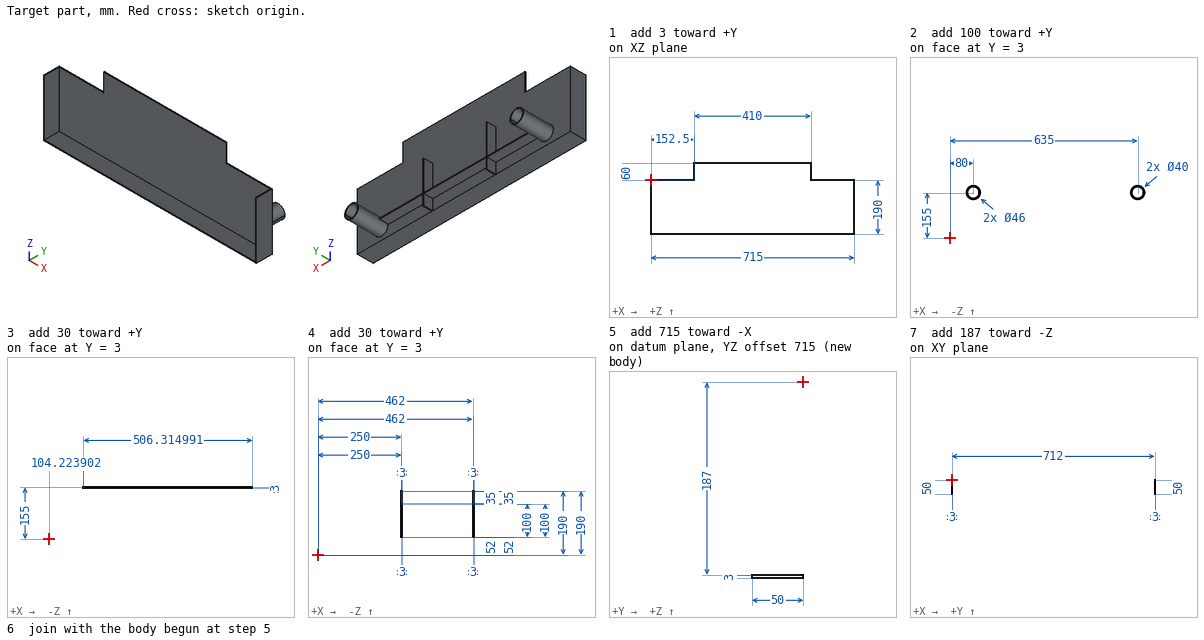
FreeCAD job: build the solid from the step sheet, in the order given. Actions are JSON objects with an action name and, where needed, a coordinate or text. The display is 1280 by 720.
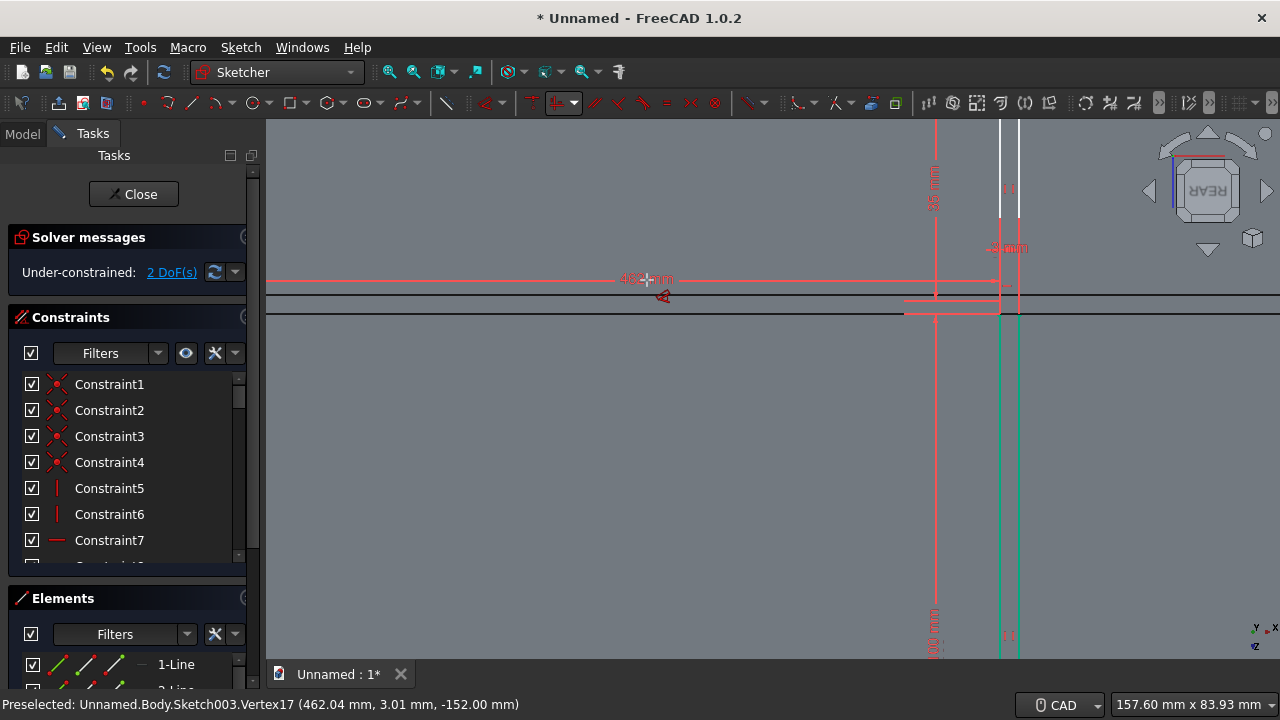
{"action": "scroll", "coordinate": [1003, 315], "scroll_direction": "down", "scroll_amount": 8}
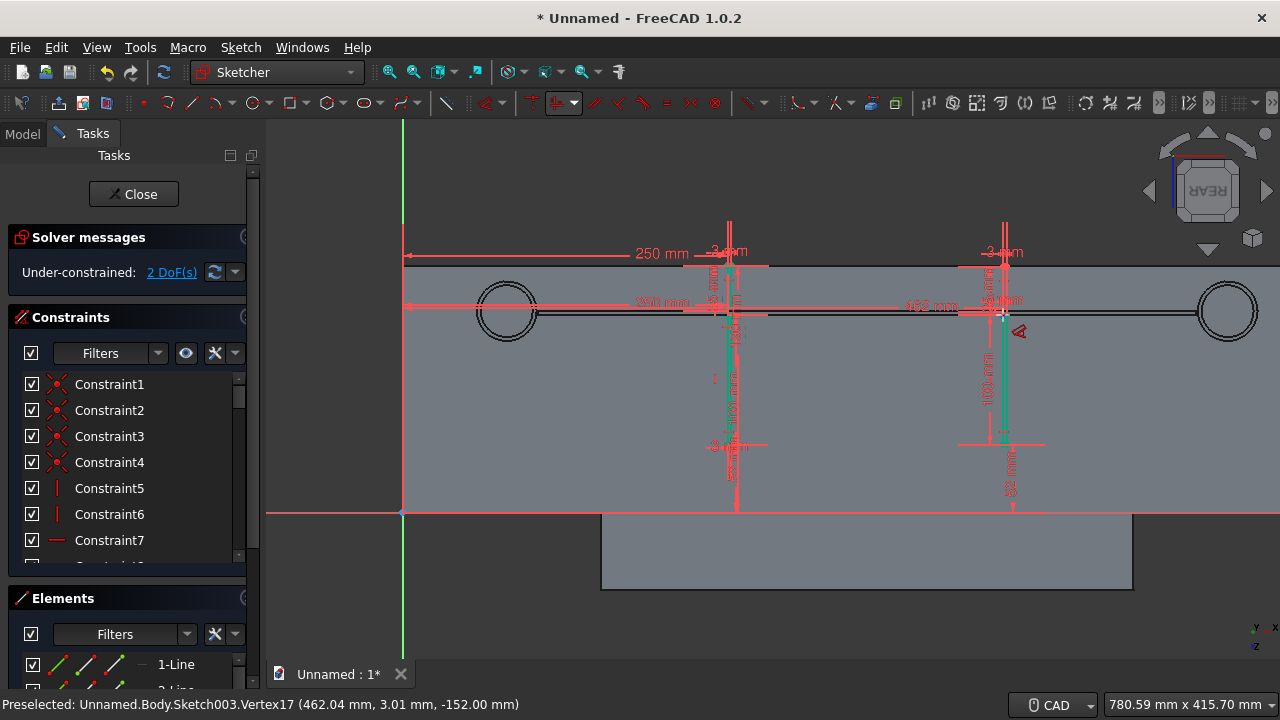
{"action": "scroll", "coordinate": [1003, 267], "scroll_direction": "up", "scroll_amount": 6}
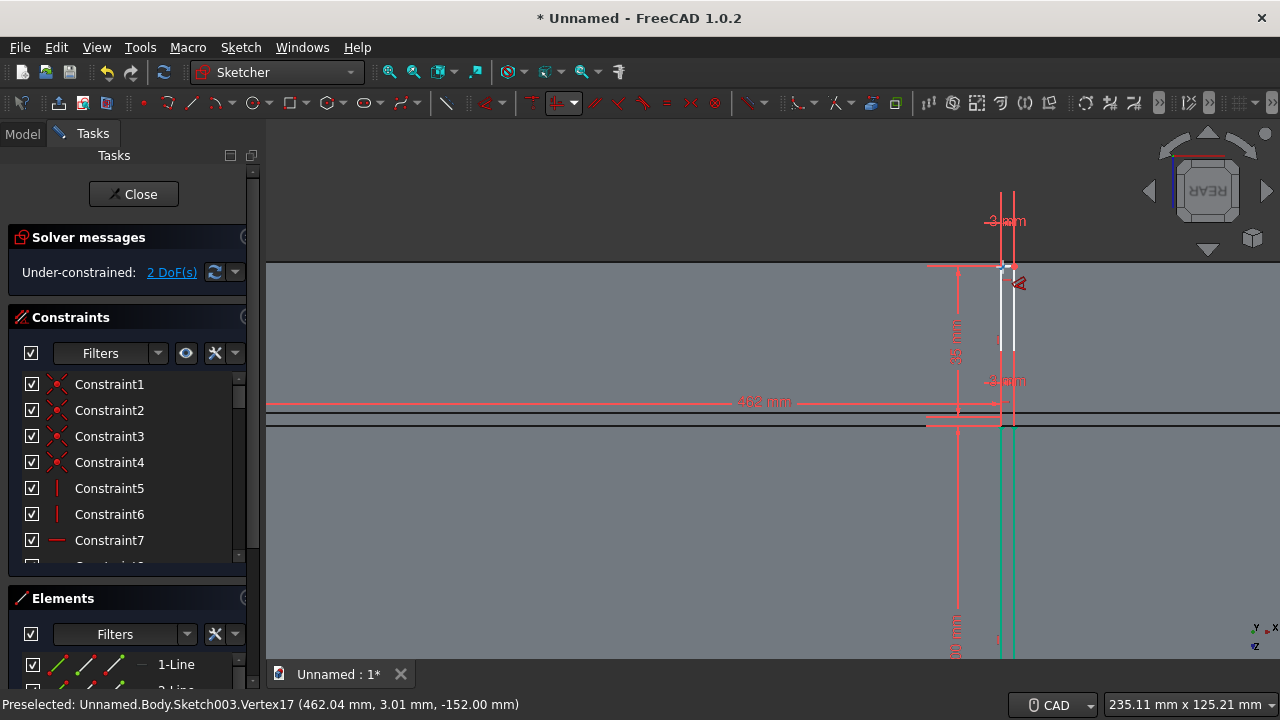
{"action": "left_click", "coordinate": [1001, 266]}
{"action": "left_click", "coordinate": [648, 232]}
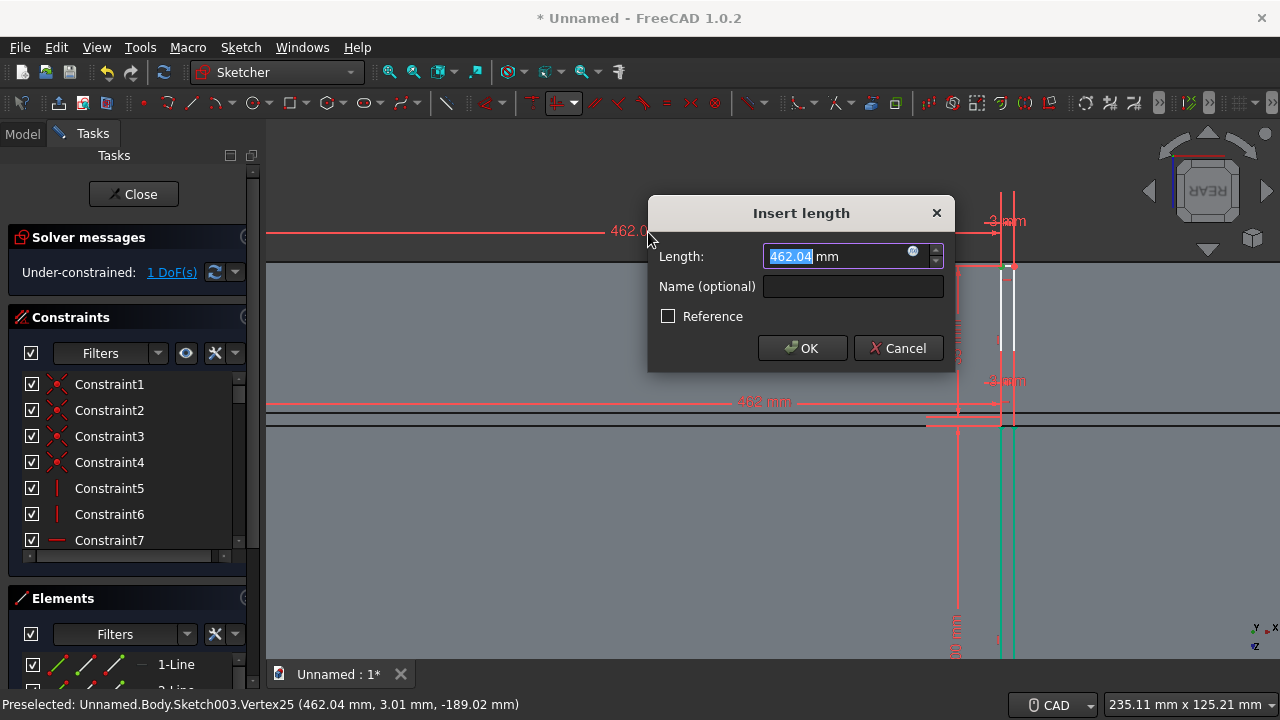
{"action": "type", "text": "462"}
{"action": "key", "text": "Return"}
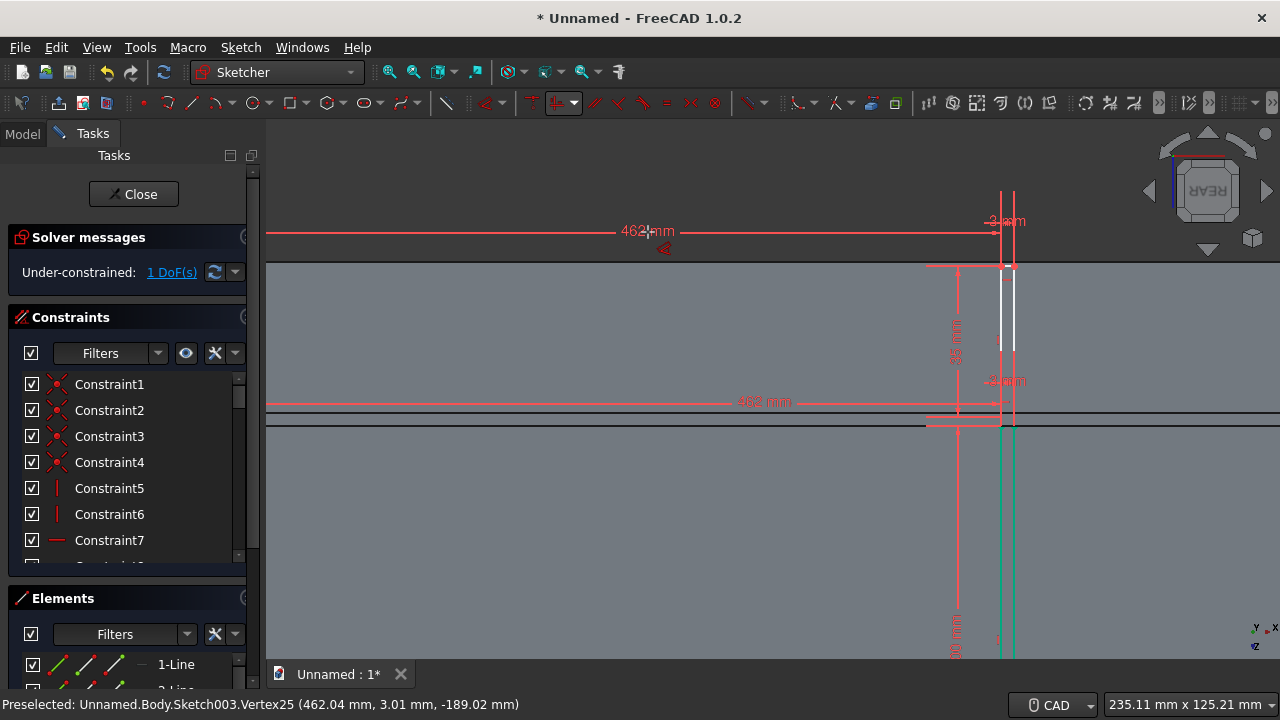
{"action": "left_click", "coordinate": [1001, 266]}
{"action": "left_click", "coordinate": [1035, 449]}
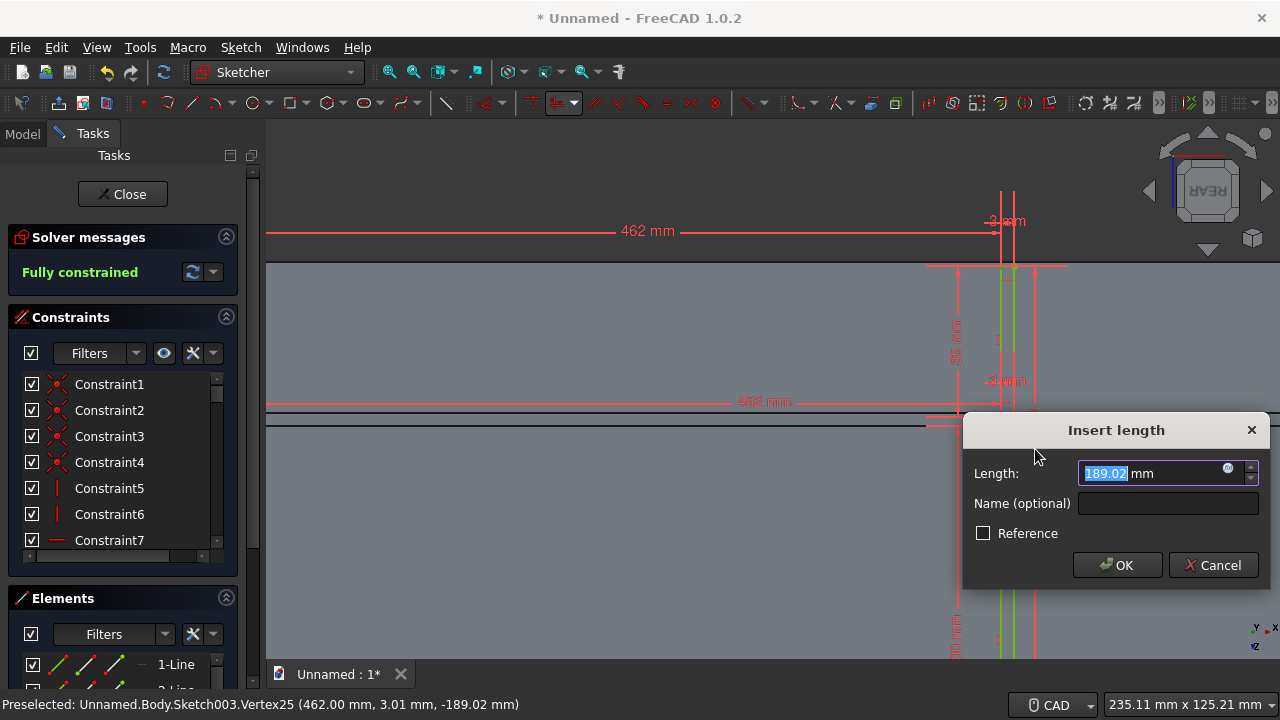
{"action": "type", "text": "190"}
{"action": "key", "text": "Return"}
{"action": "key", "text": "Escape"}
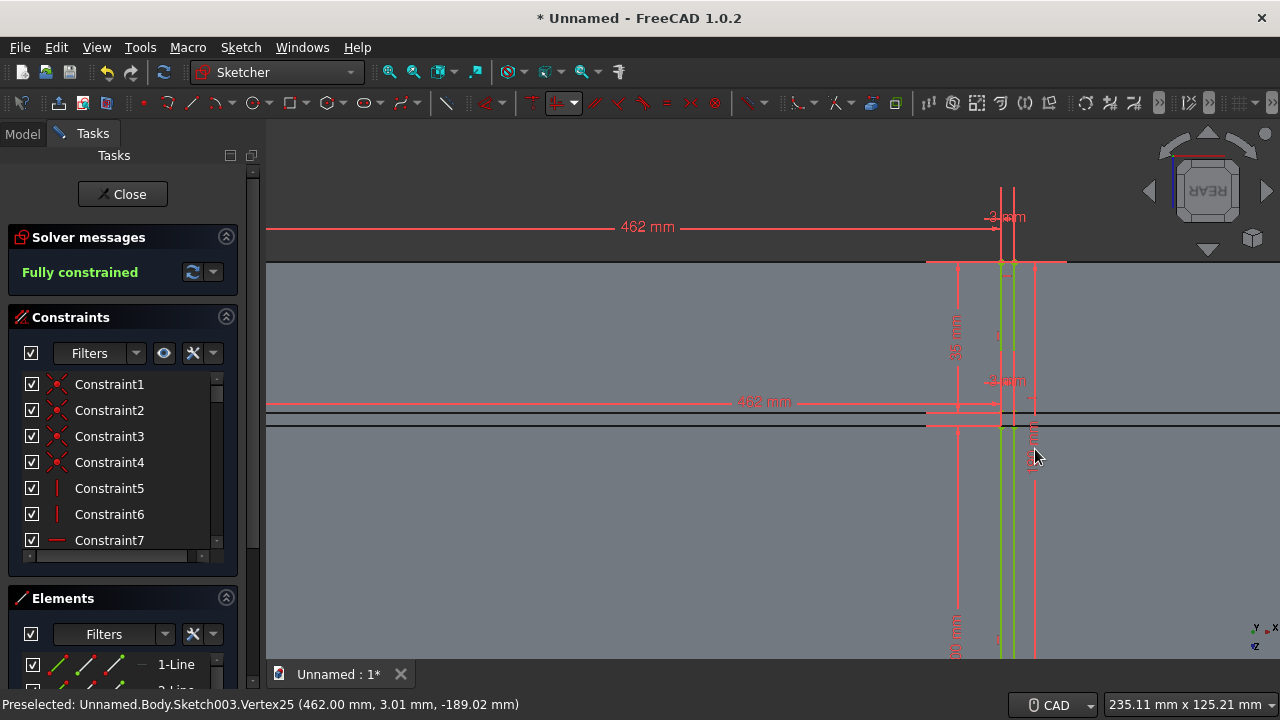
{"action": "left_click", "coordinate": [123, 194]}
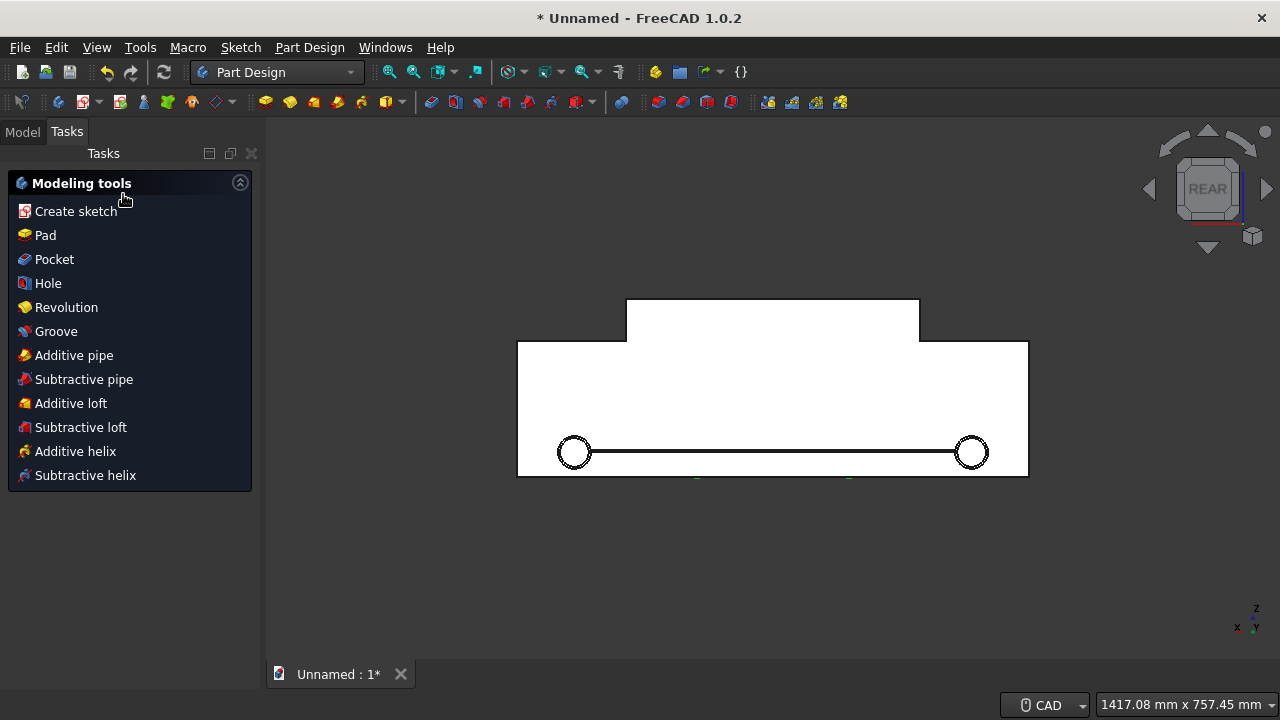
{"action": "left_click", "coordinate": [266, 102]}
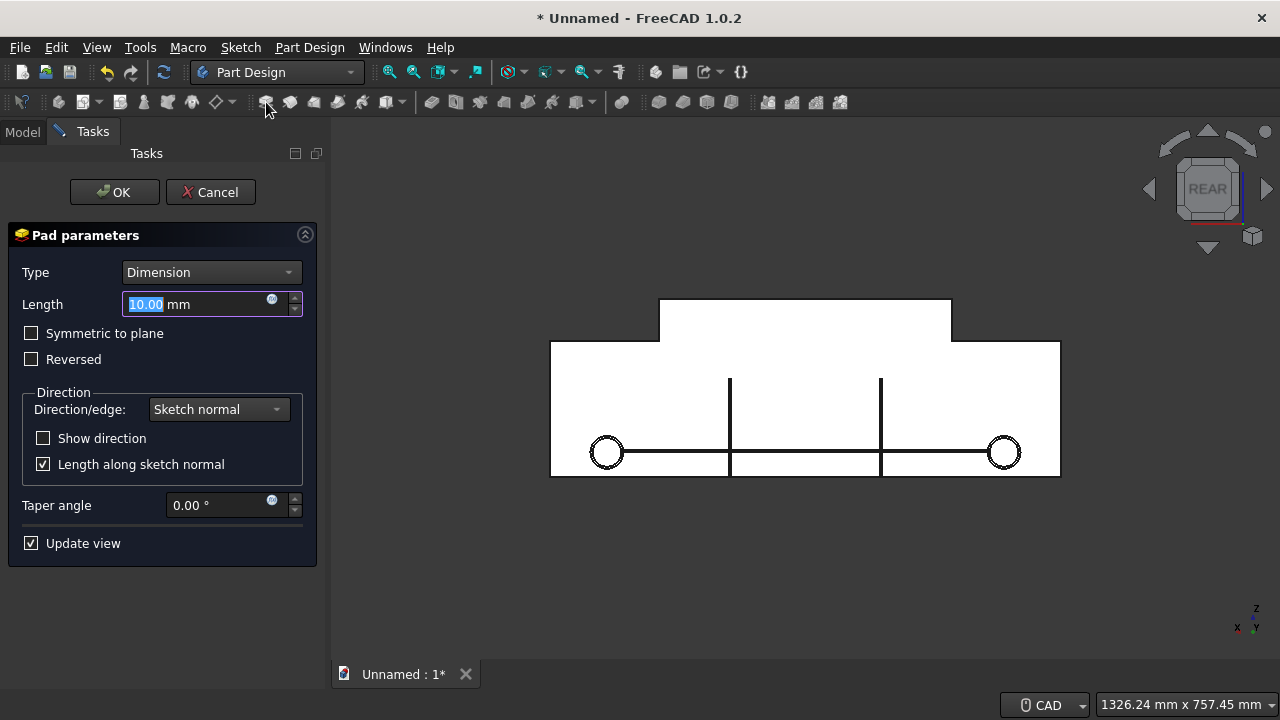
{"action": "type", "text": "30"}
{"action": "key", "text": "Tab"}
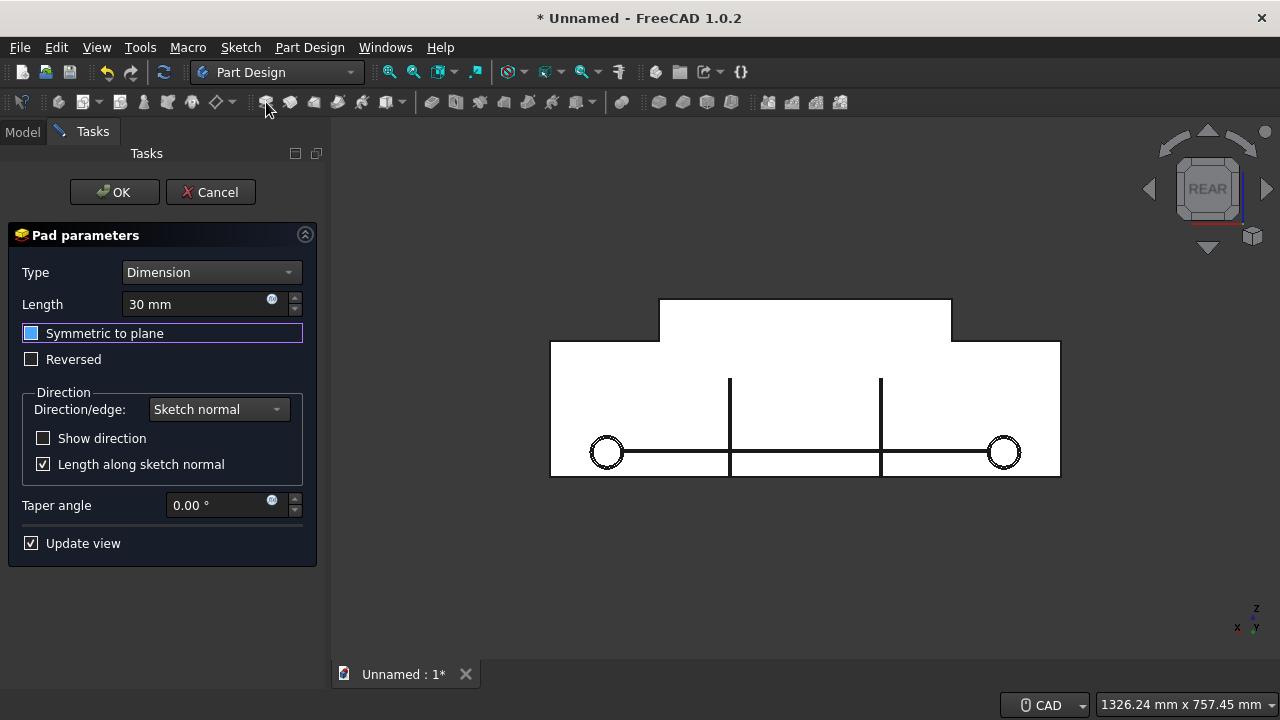
{"action": "left_click", "coordinate": [115, 192]}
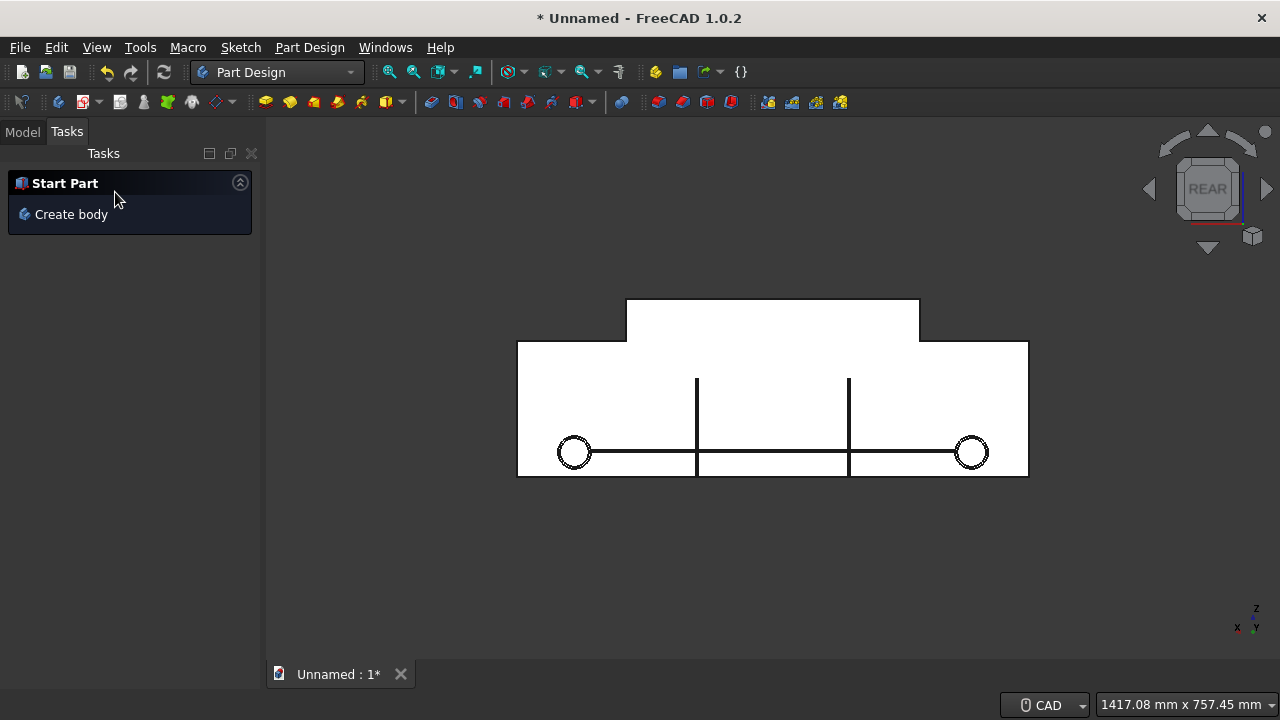
{"action": "left_click", "coordinate": [60, 102]}